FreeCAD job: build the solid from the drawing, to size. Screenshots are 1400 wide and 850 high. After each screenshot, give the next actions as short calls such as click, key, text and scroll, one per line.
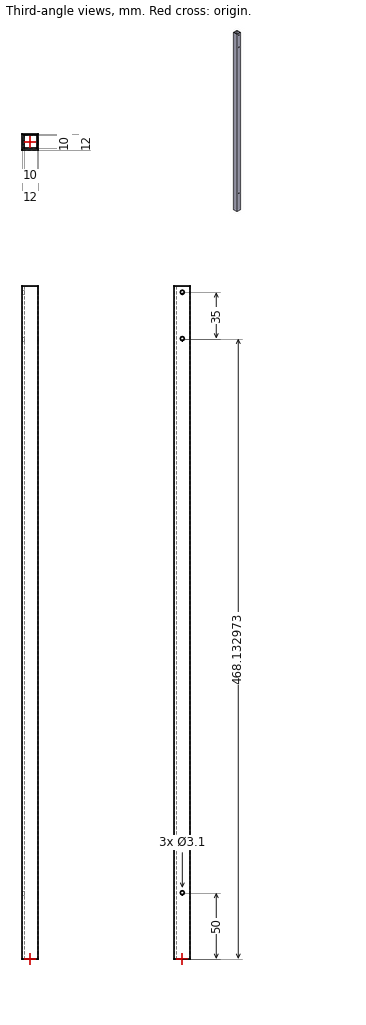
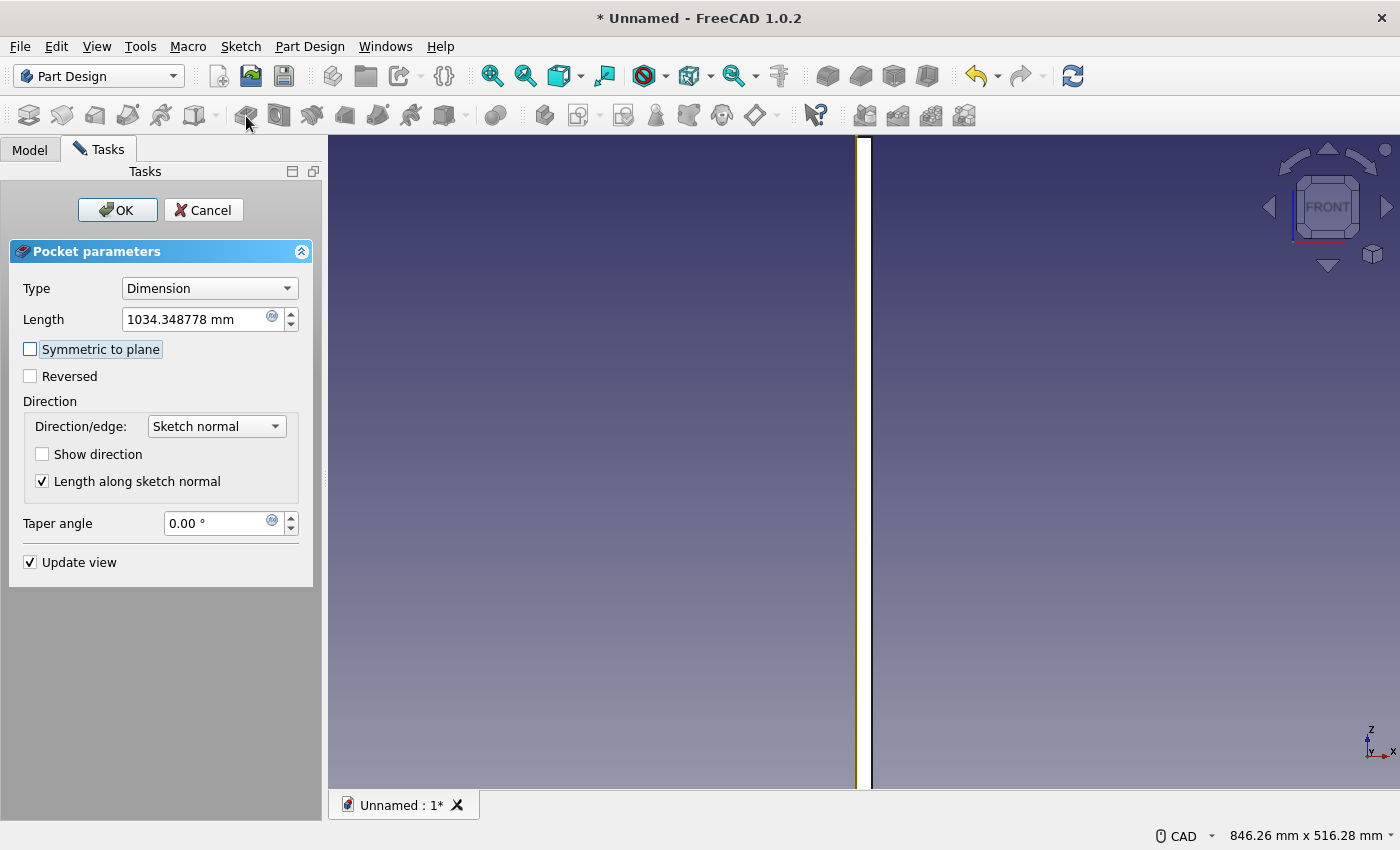
click(31, 349)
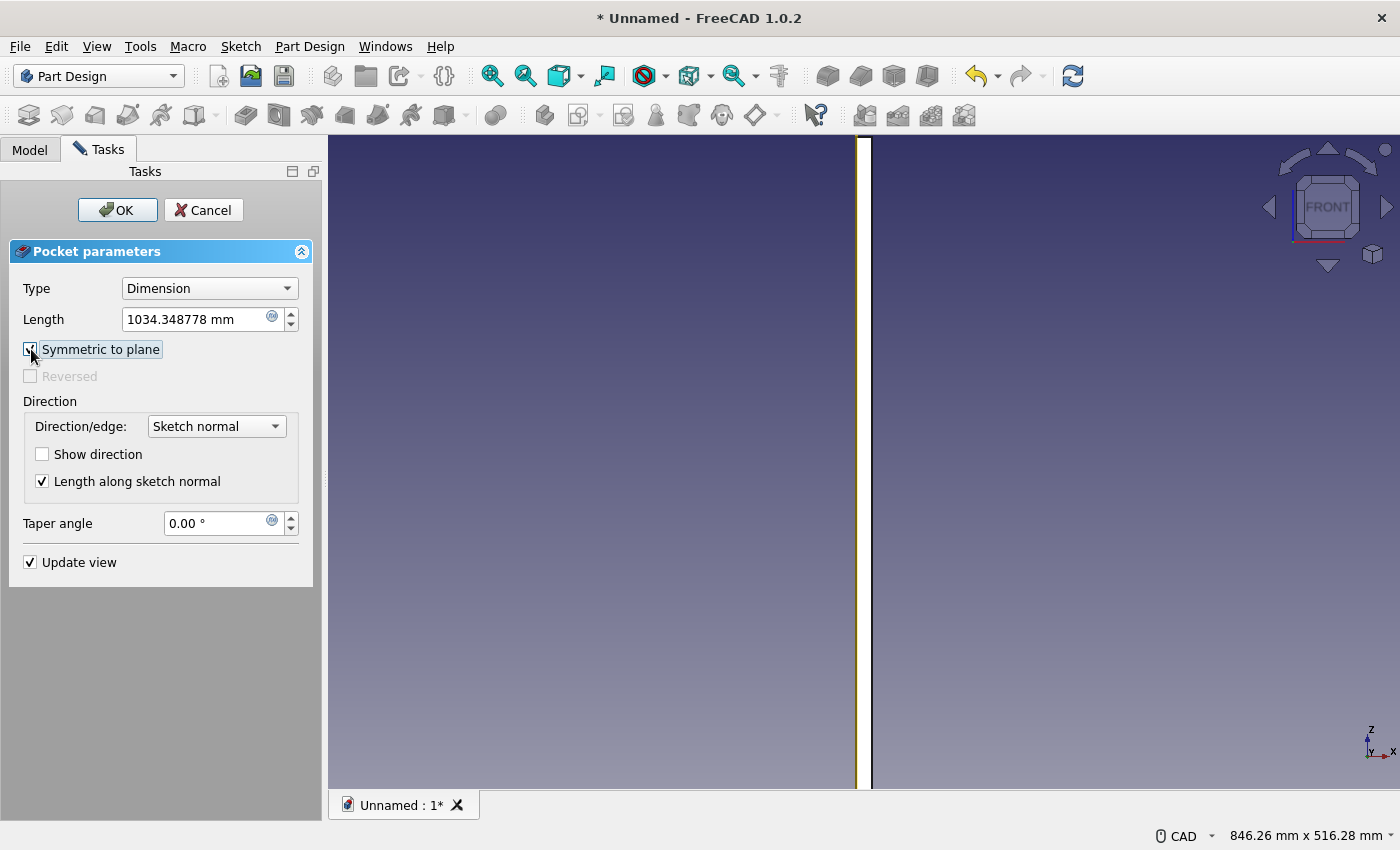
click(118, 210)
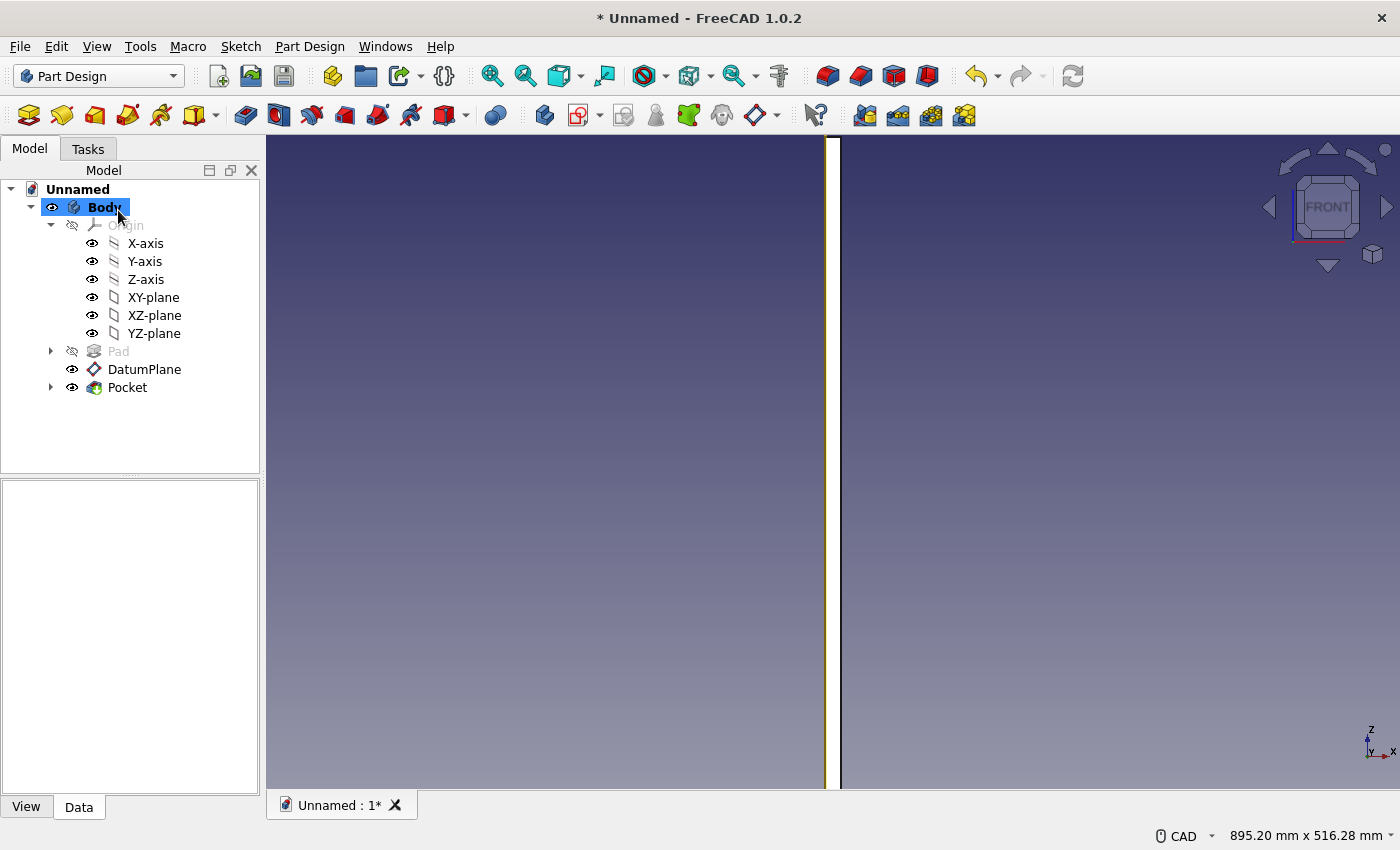
click(117, 369)
key(space)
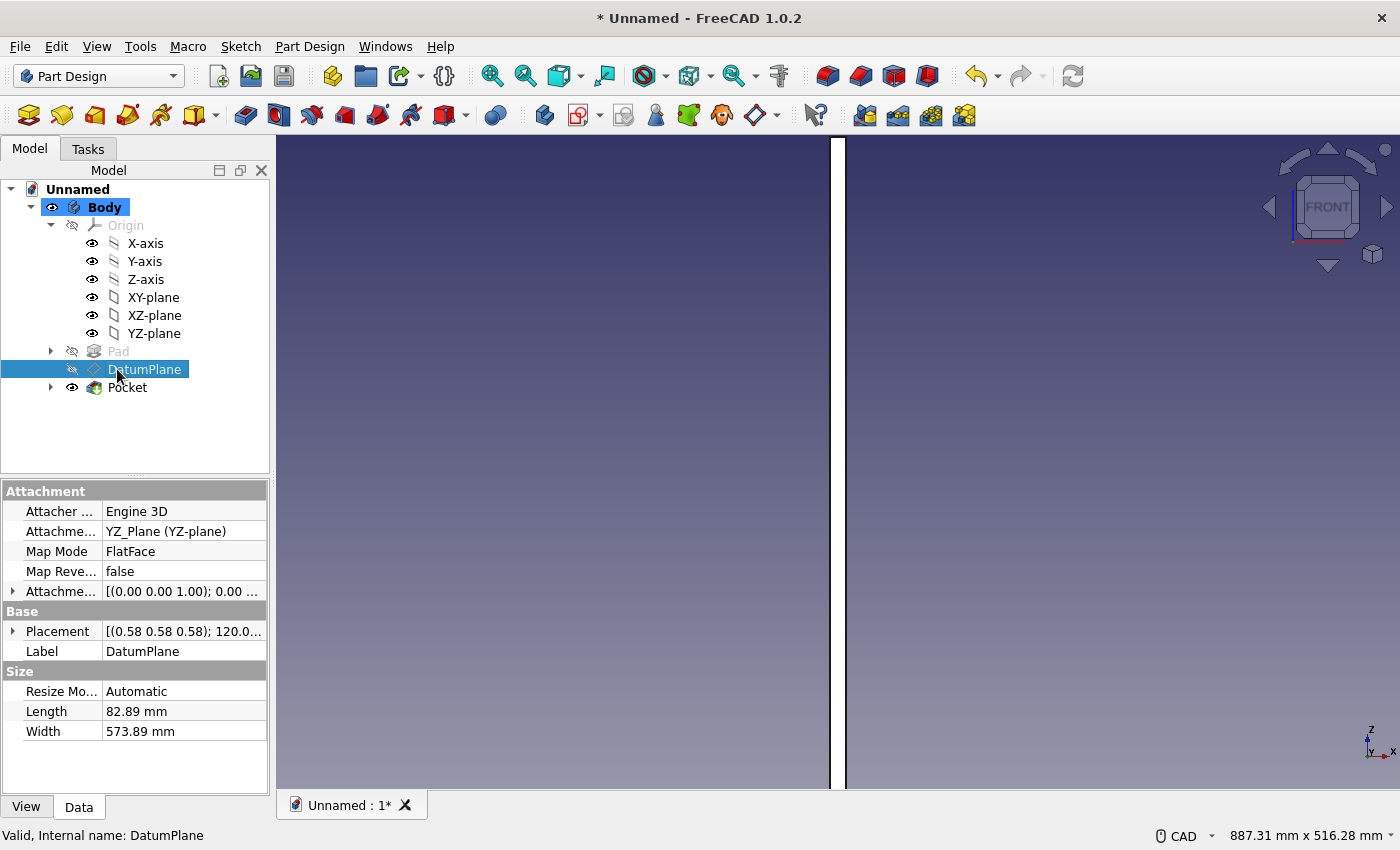
click(493, 76)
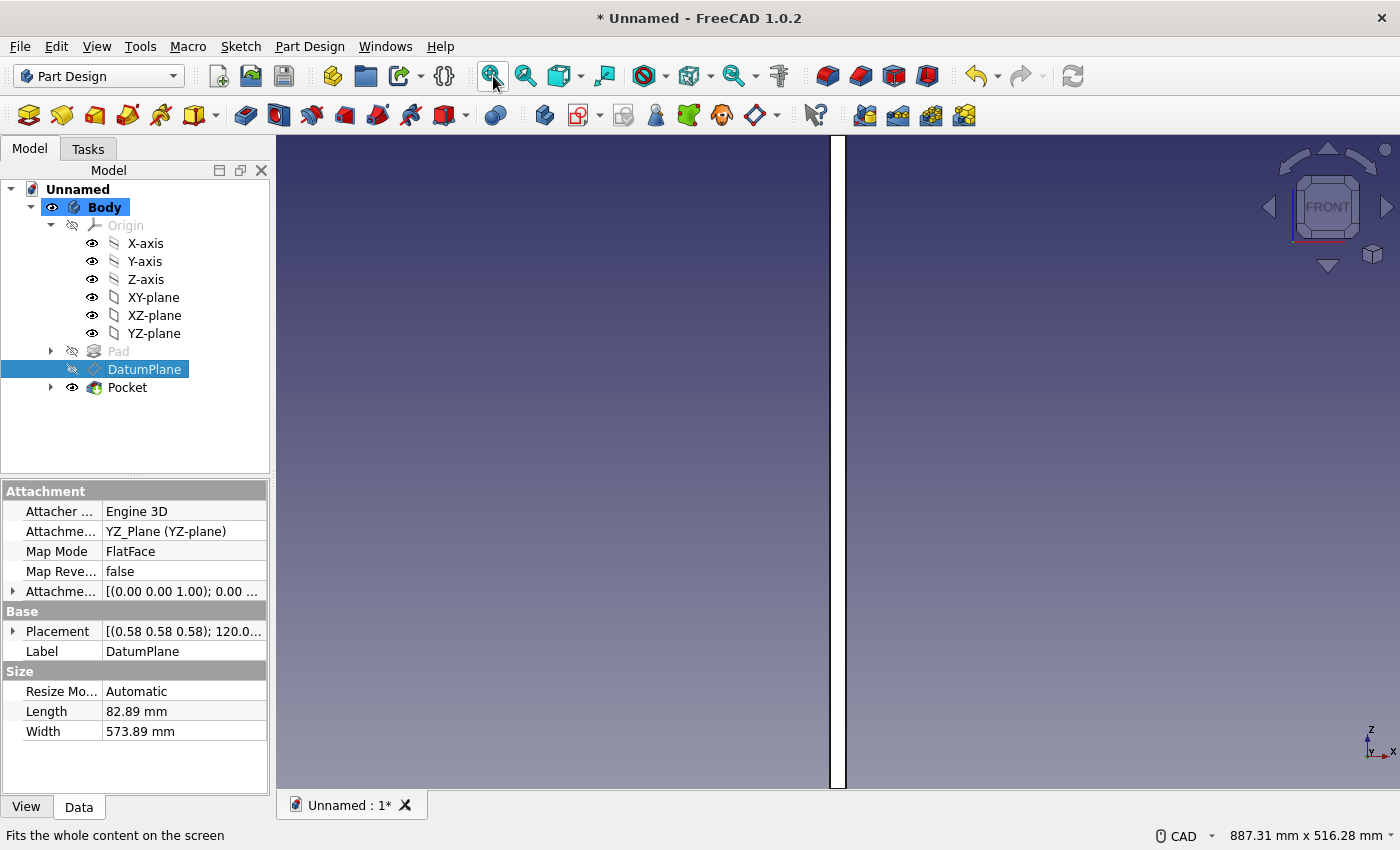
key(0)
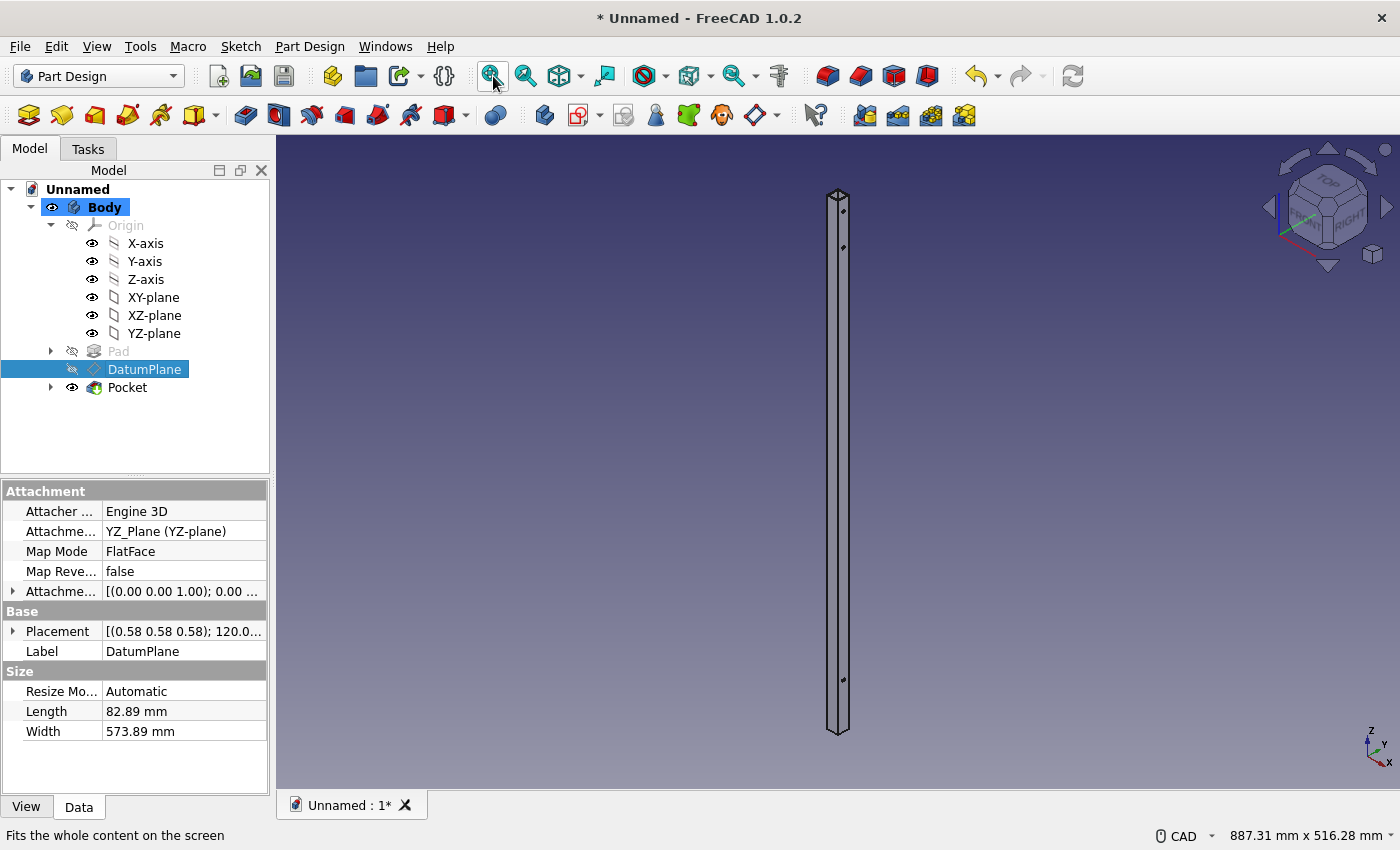
scroll(829, 194, up, 15)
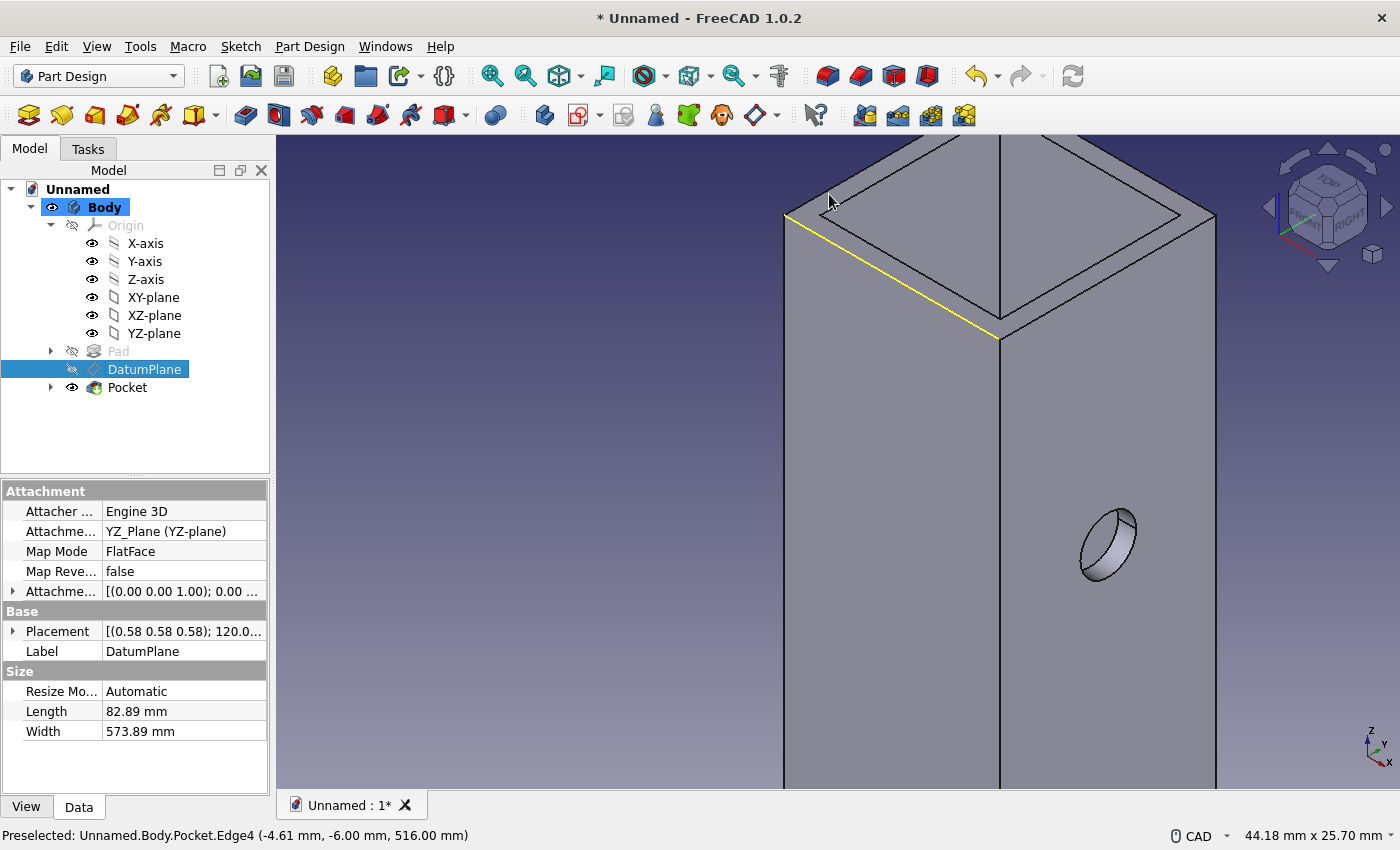
scroll(815, 214, up, 5)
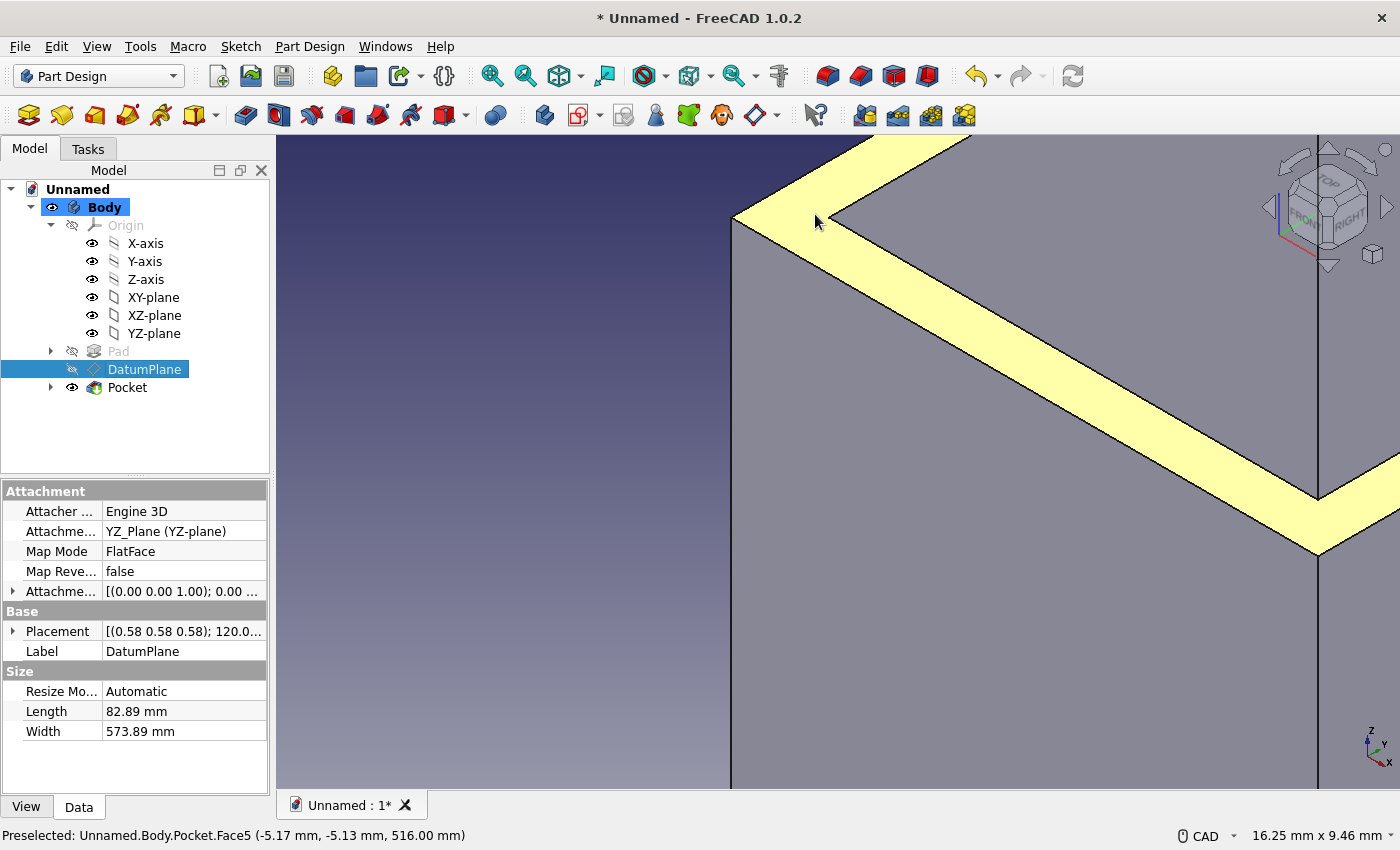
click(815, 217)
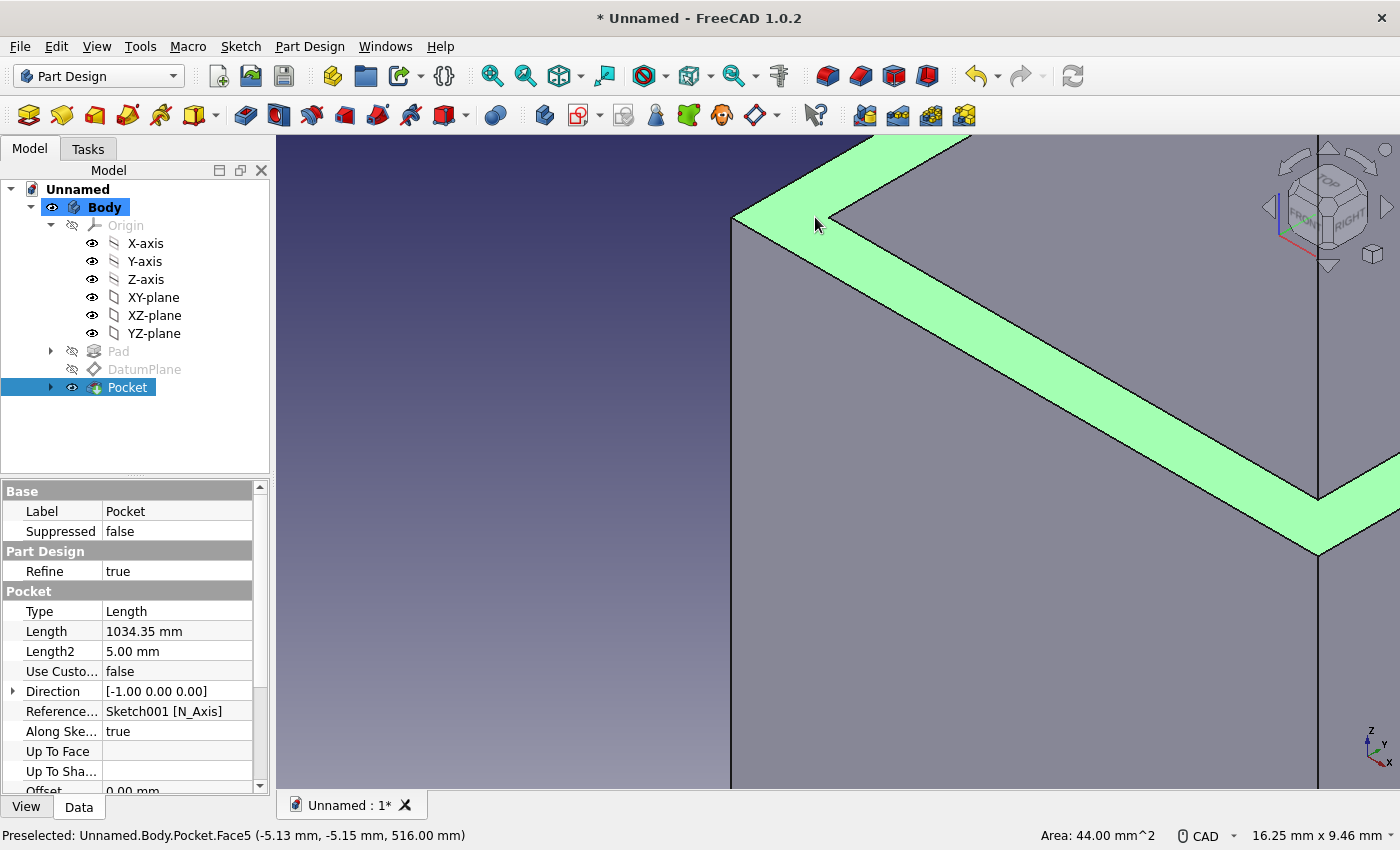
click(578, 116)